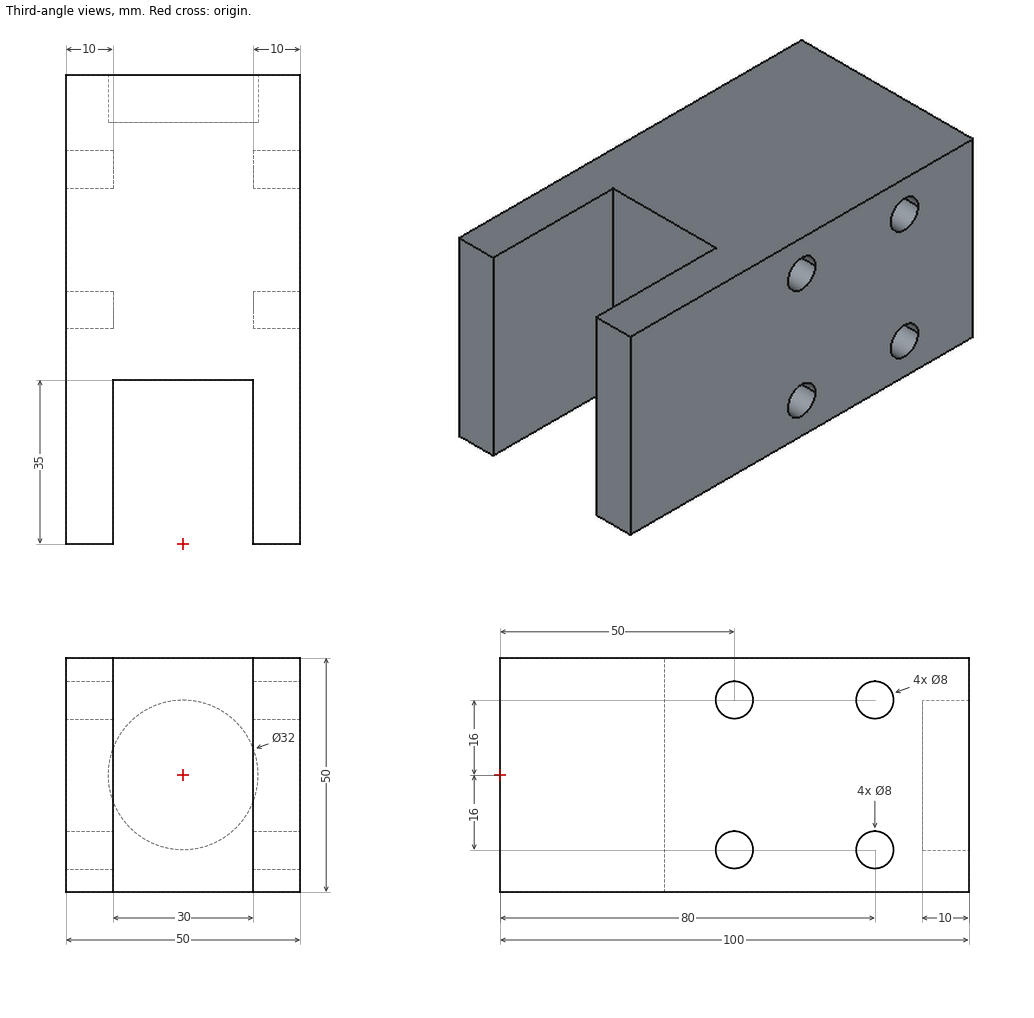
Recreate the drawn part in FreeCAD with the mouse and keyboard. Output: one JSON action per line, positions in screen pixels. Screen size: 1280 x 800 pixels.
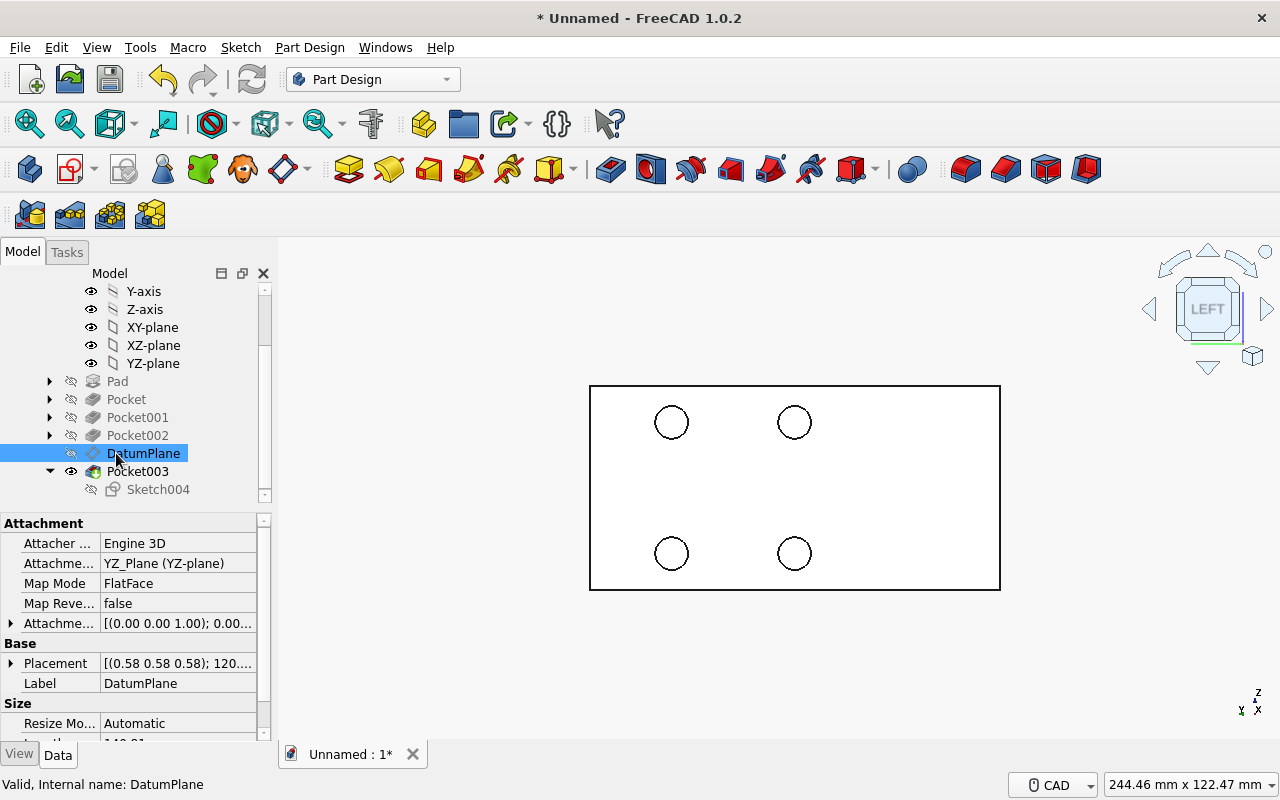
{"action": "key", "text": "0"}